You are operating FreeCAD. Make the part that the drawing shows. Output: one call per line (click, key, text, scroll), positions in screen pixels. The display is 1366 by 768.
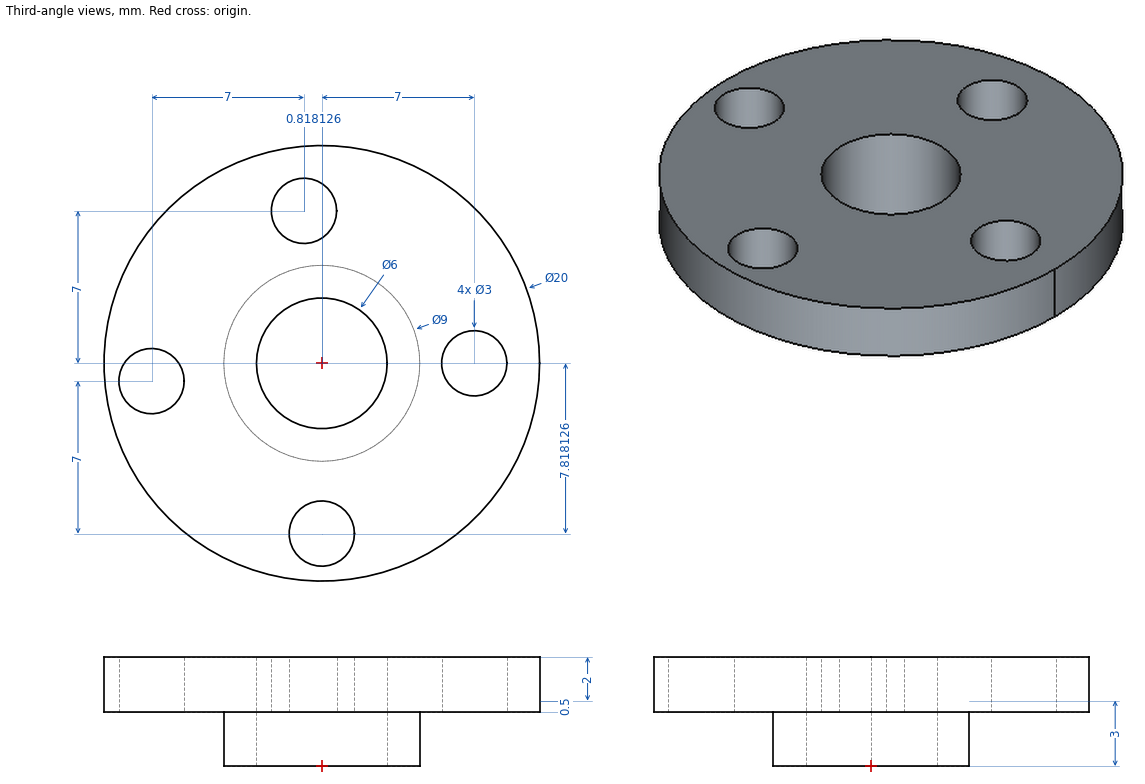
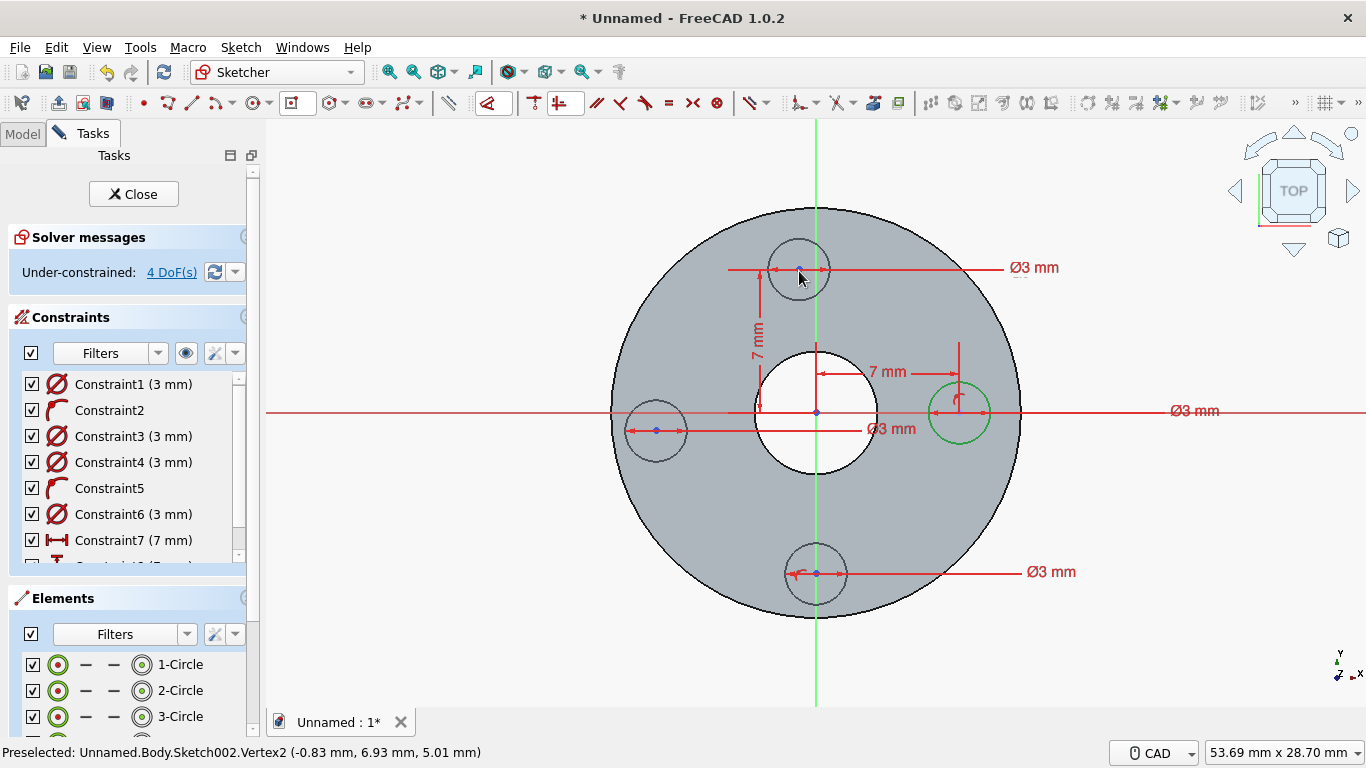
click(799, 270)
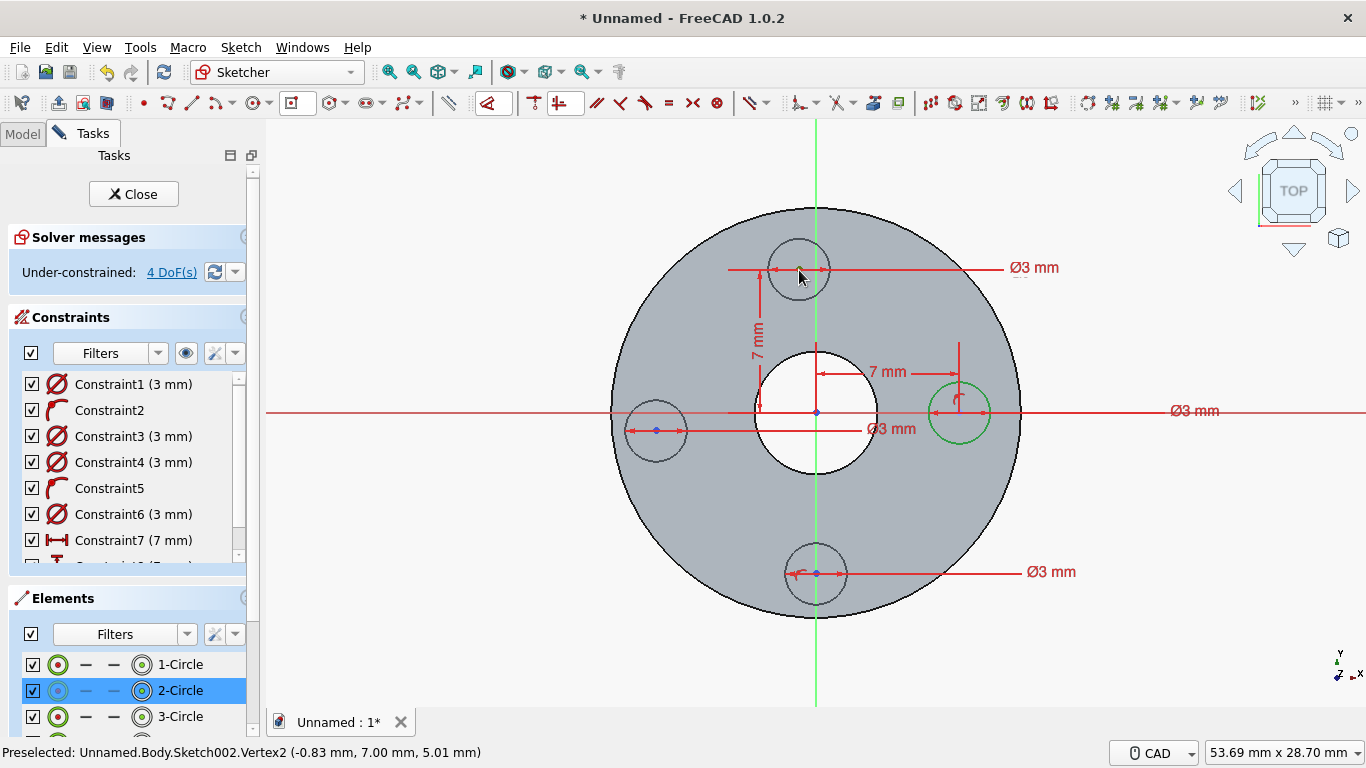
click(656, 431)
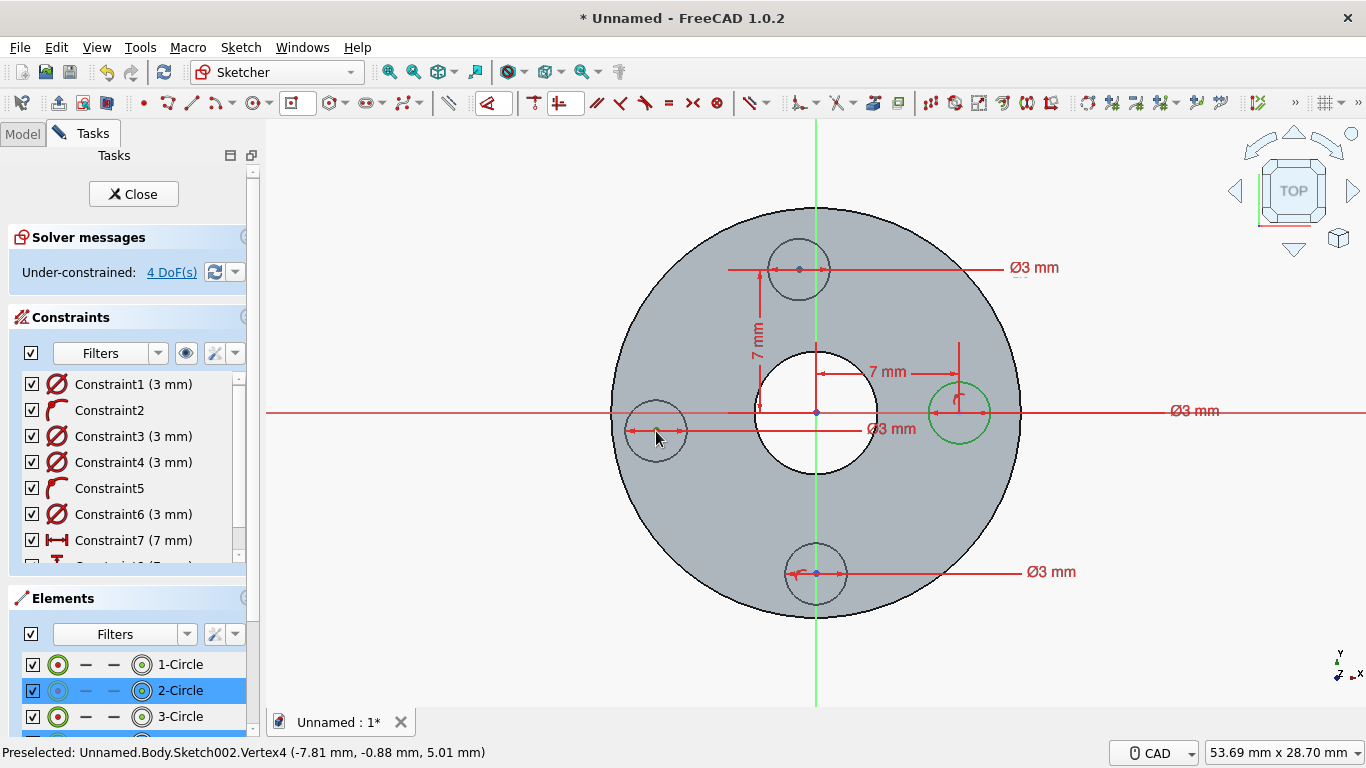
key(l)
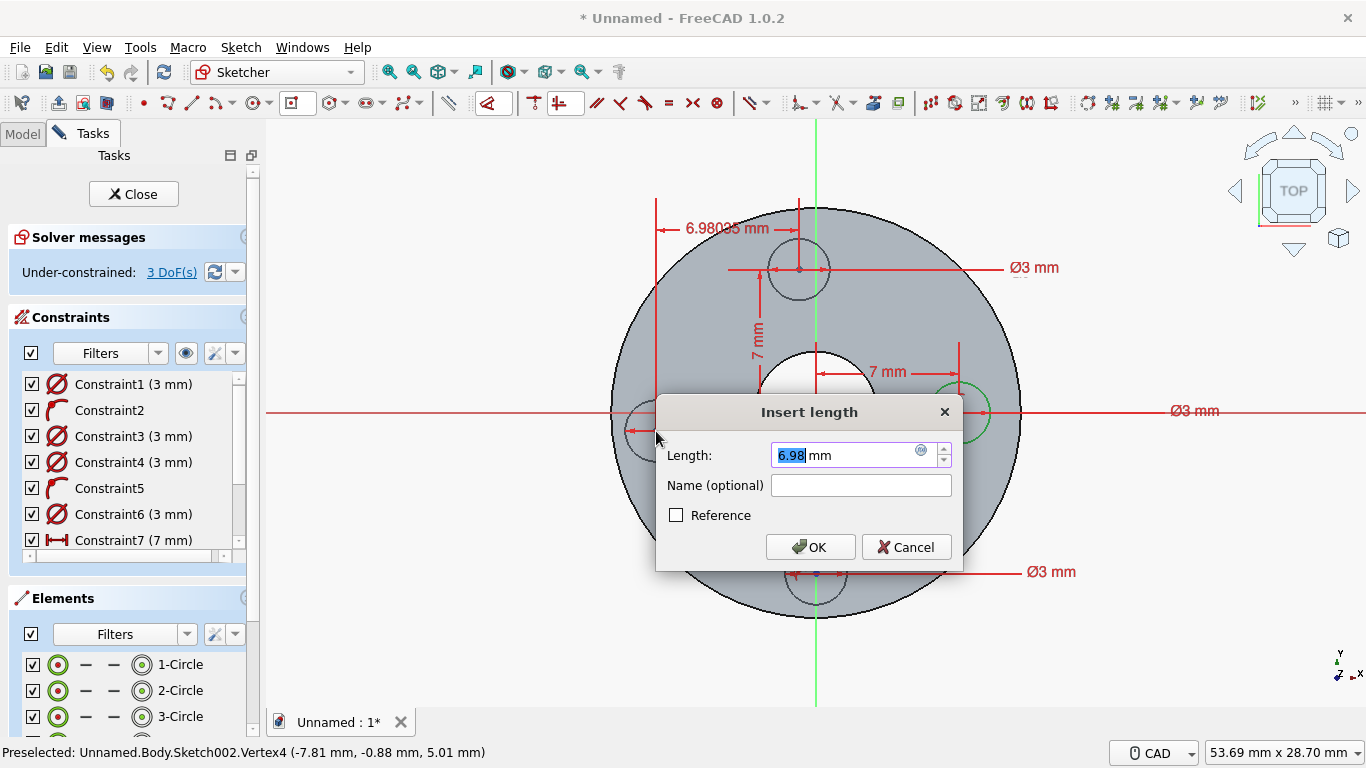
text(7)
key(Return)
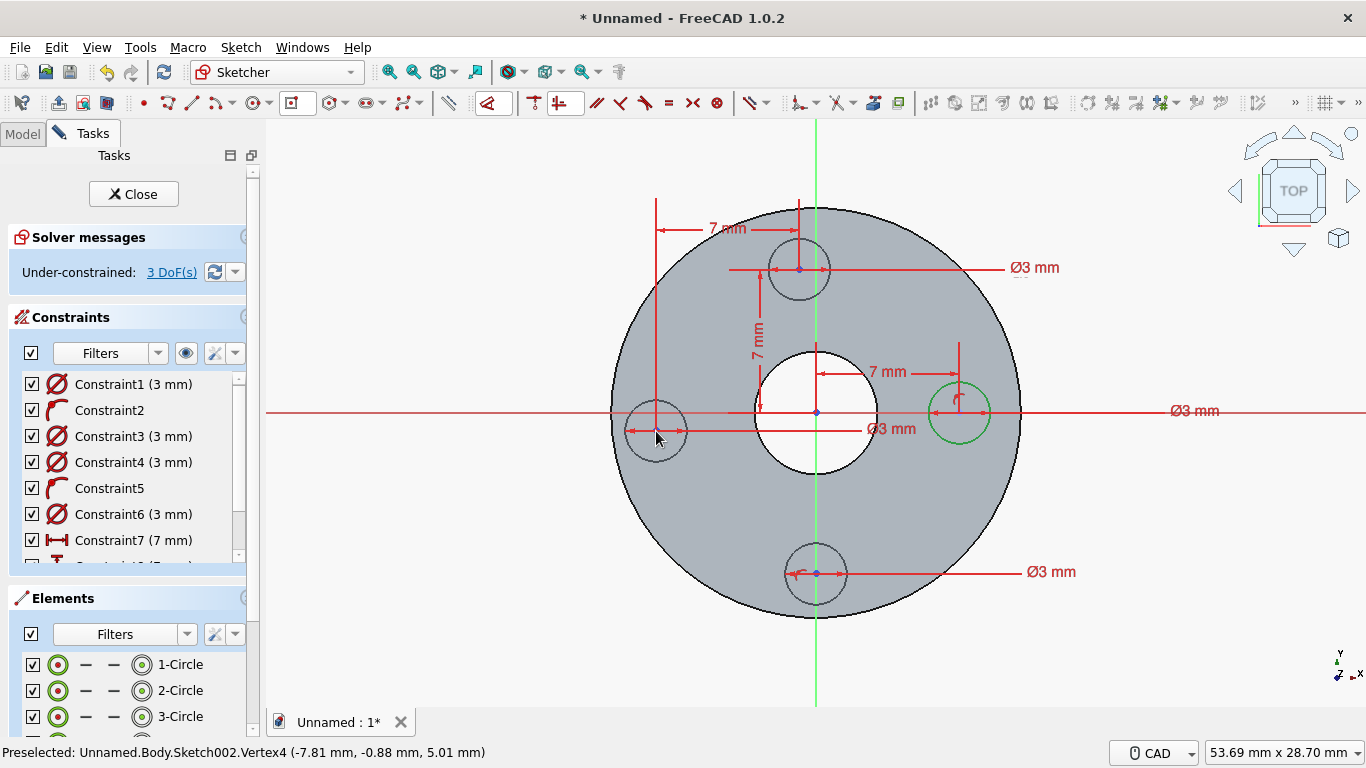
click(816, 574)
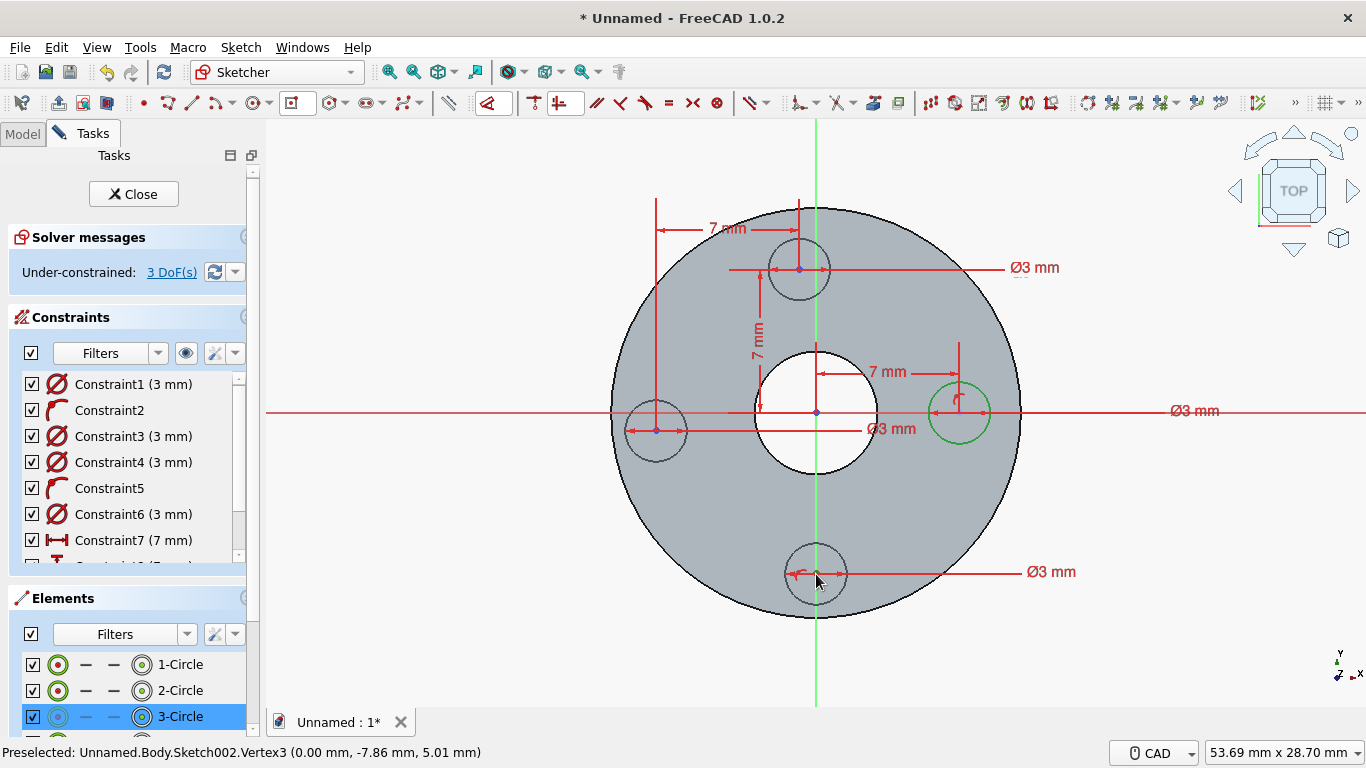
click(656, 431)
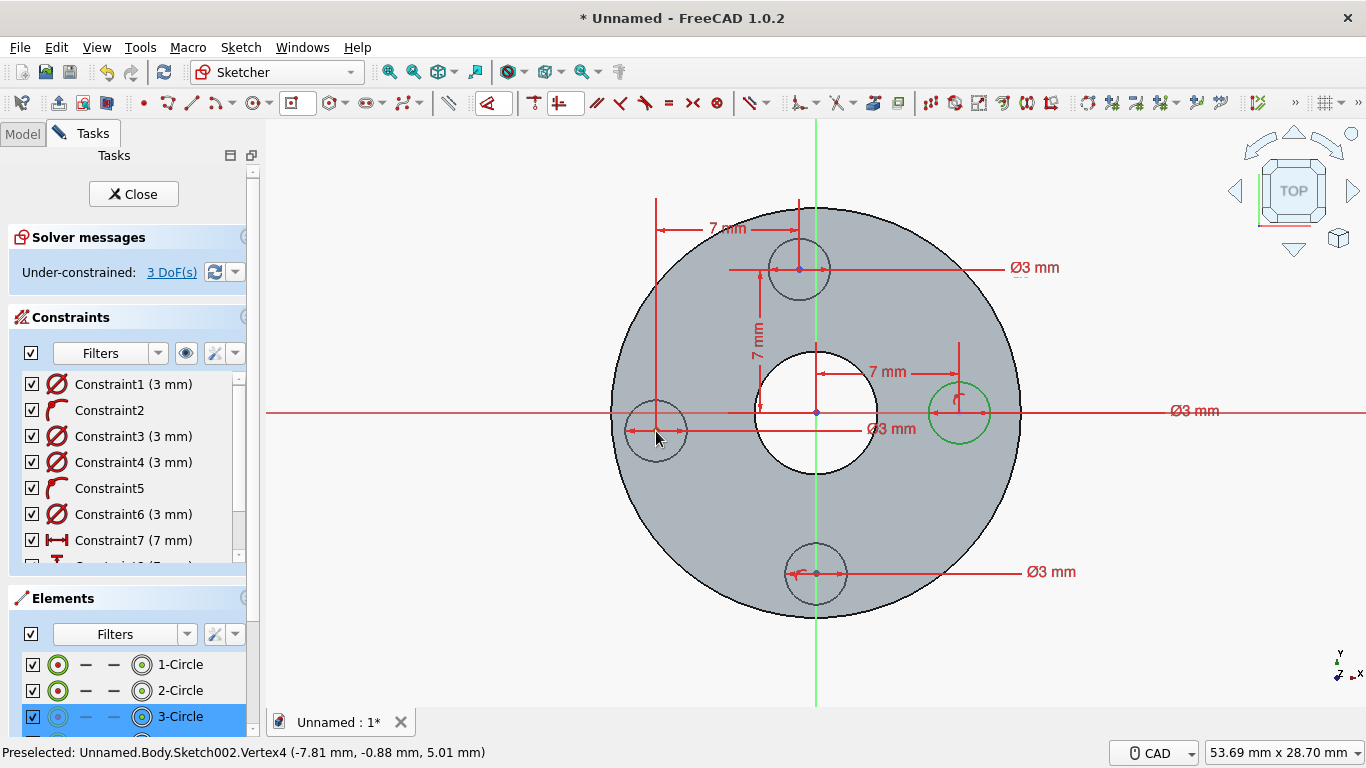
click(506, 104)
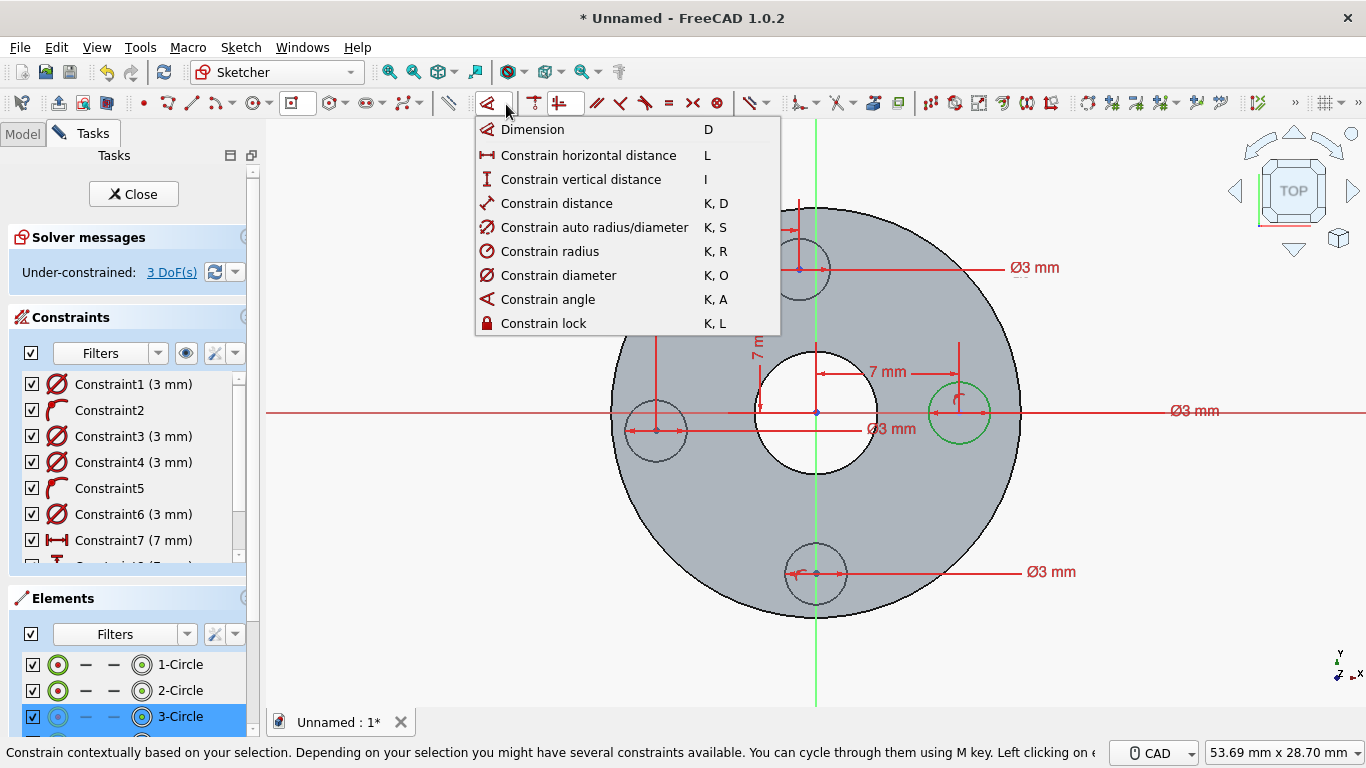
click(628, 179)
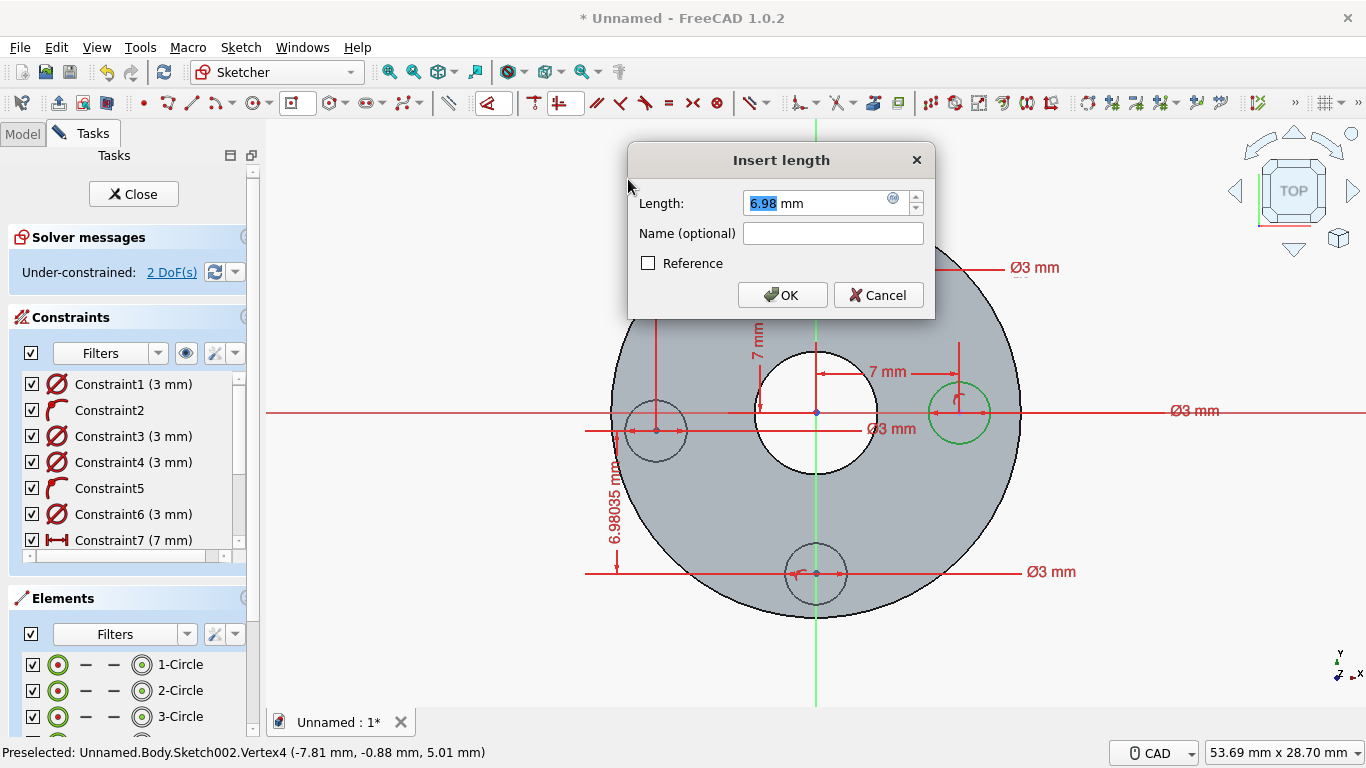
text(7)
key(Return)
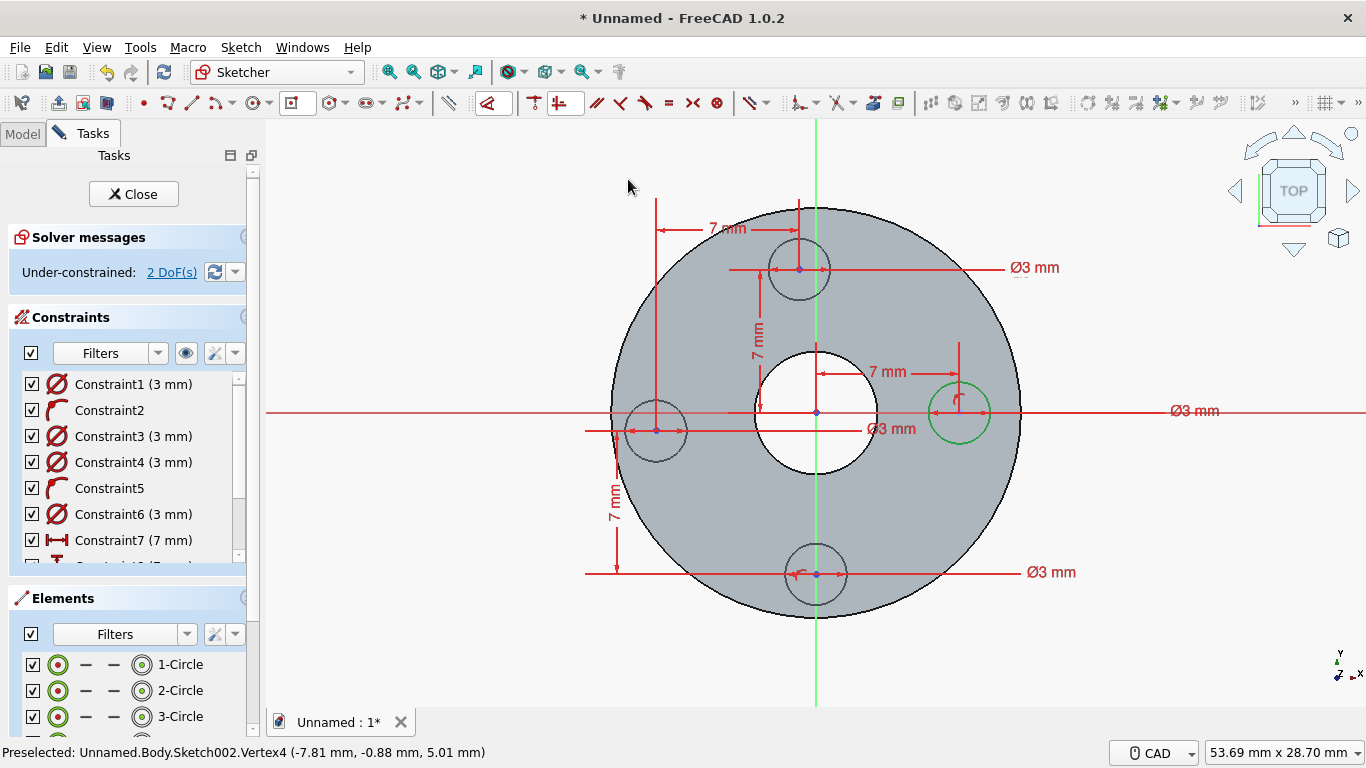
scroll(799, 270, up, 5)